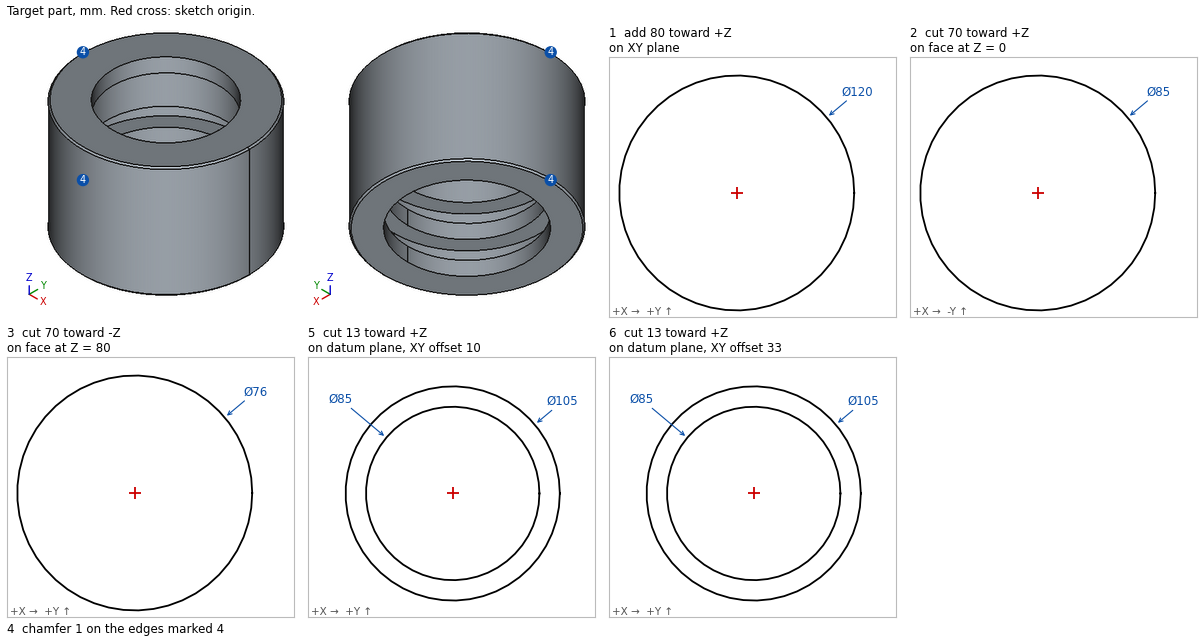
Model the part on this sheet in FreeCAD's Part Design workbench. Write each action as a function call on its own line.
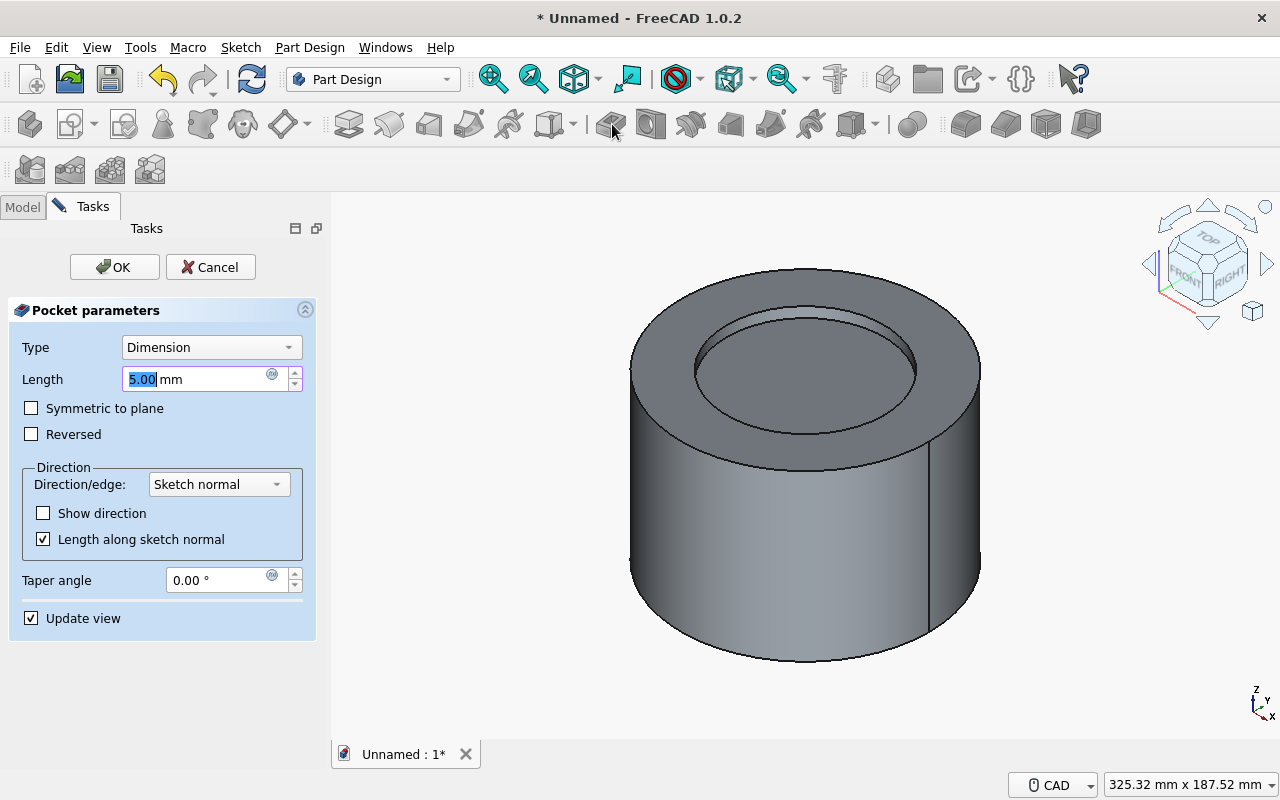
text(70)
key(Tab)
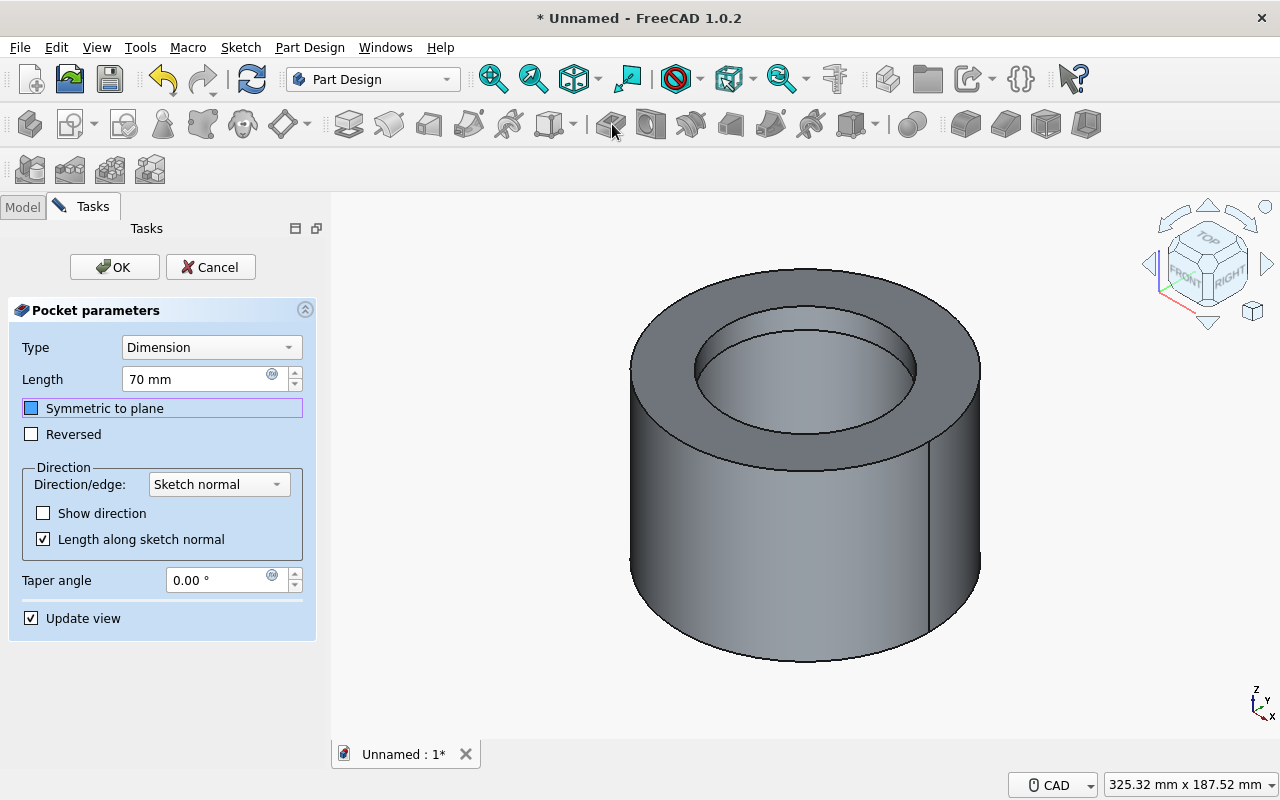
click(115, 267)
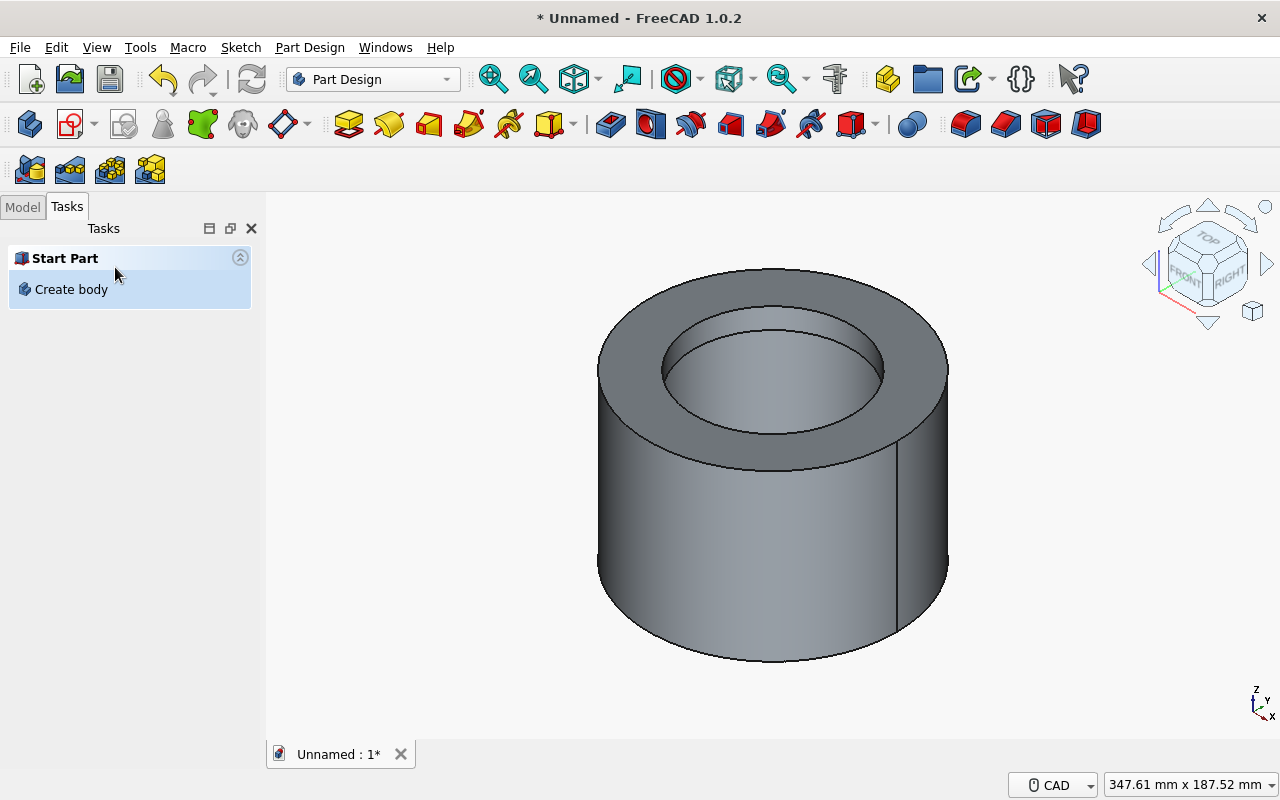
click(617, 415)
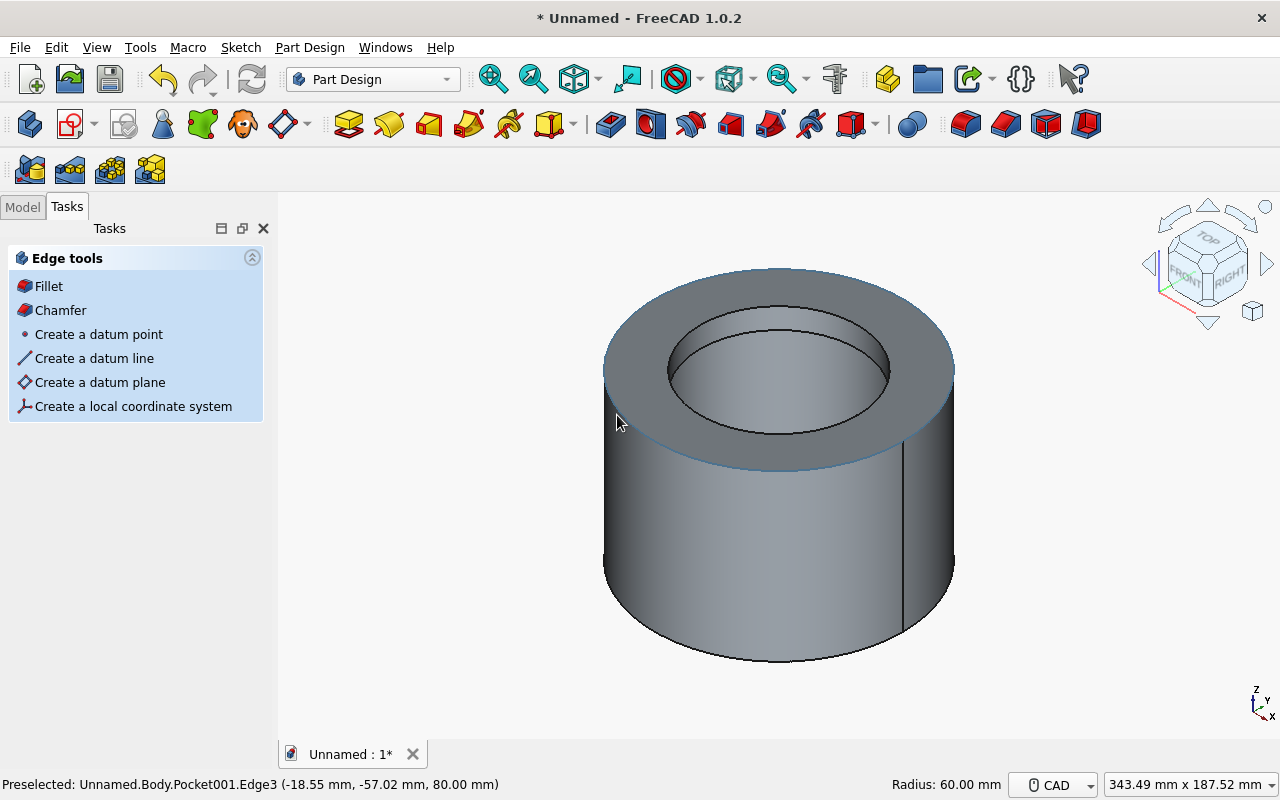
key(2)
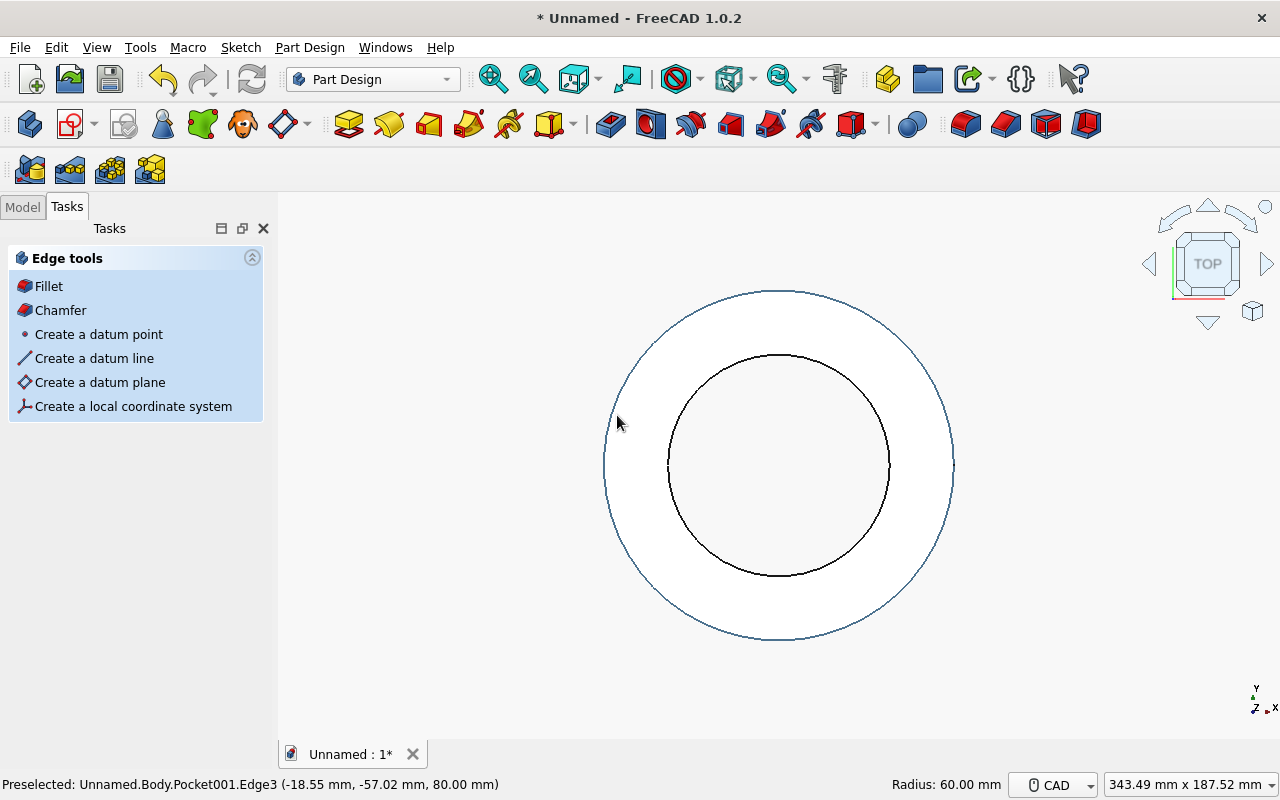
key(0)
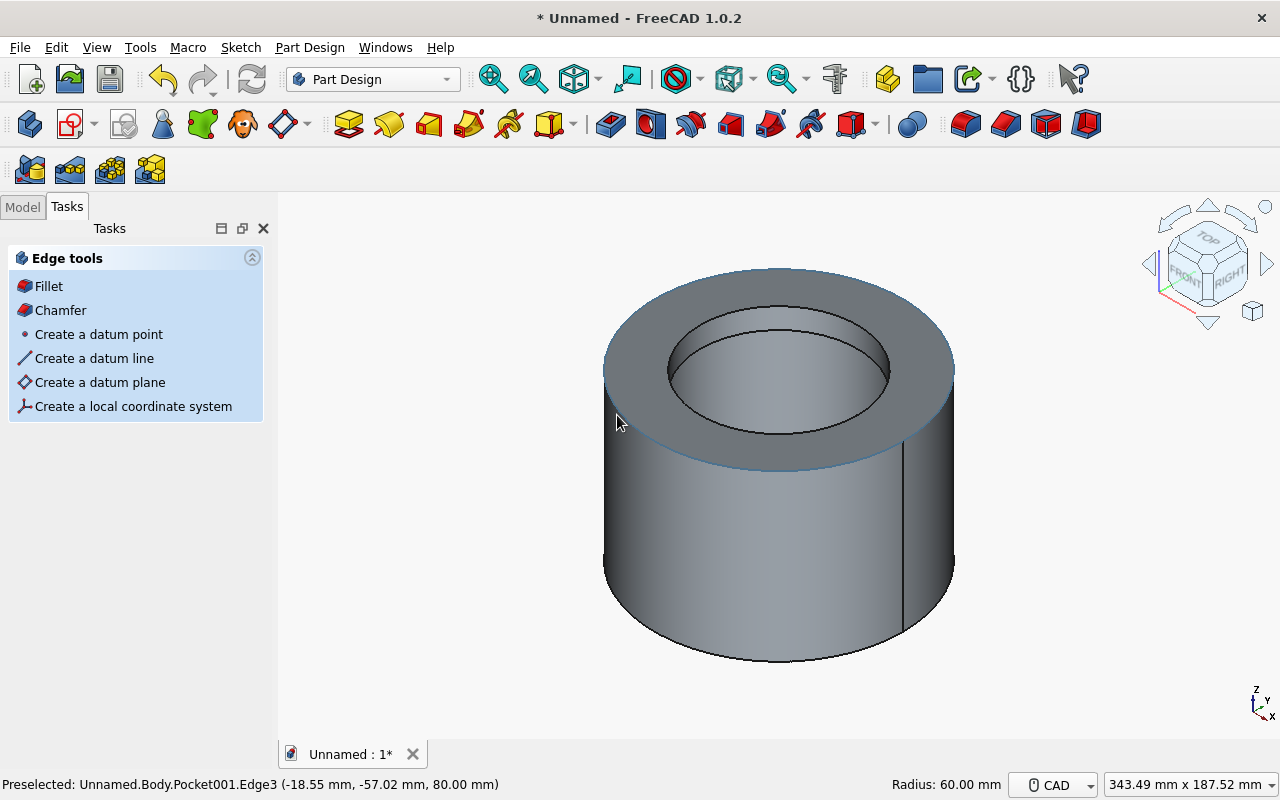
key(1)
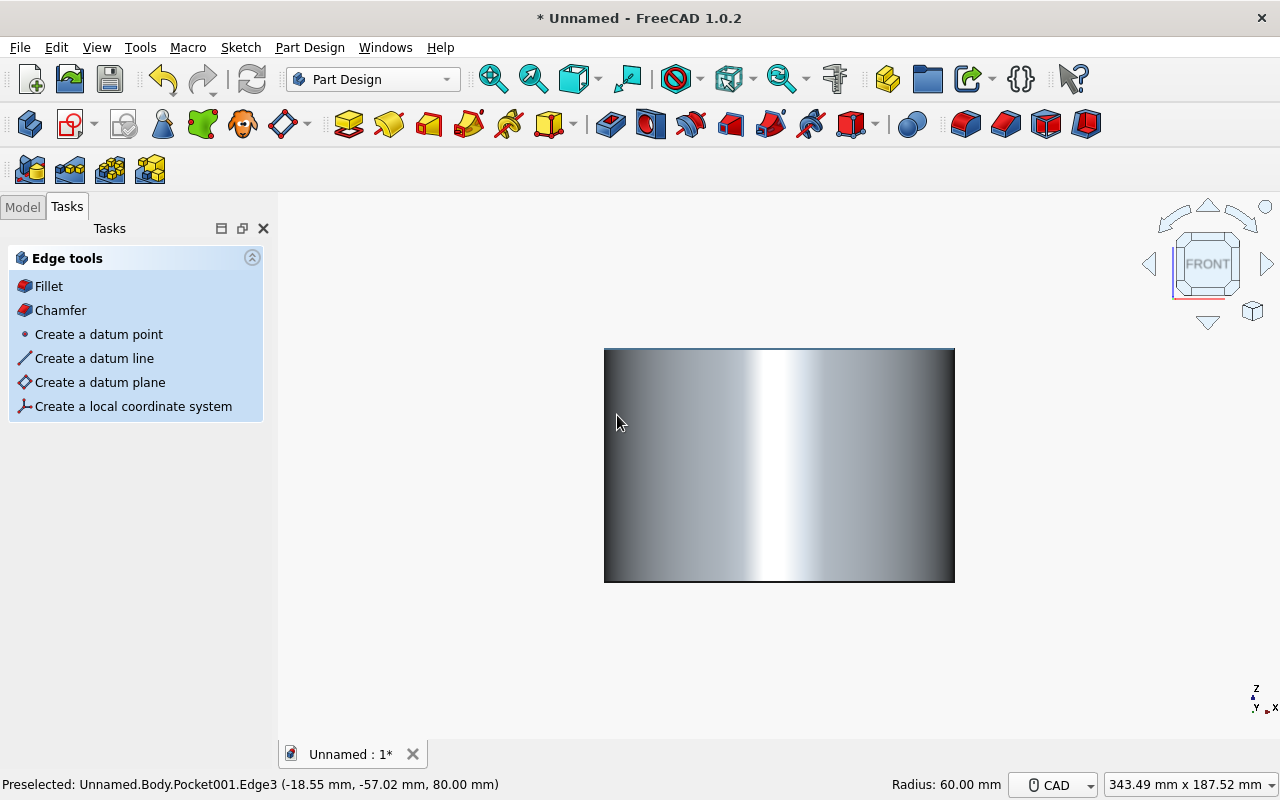
click(494, 80)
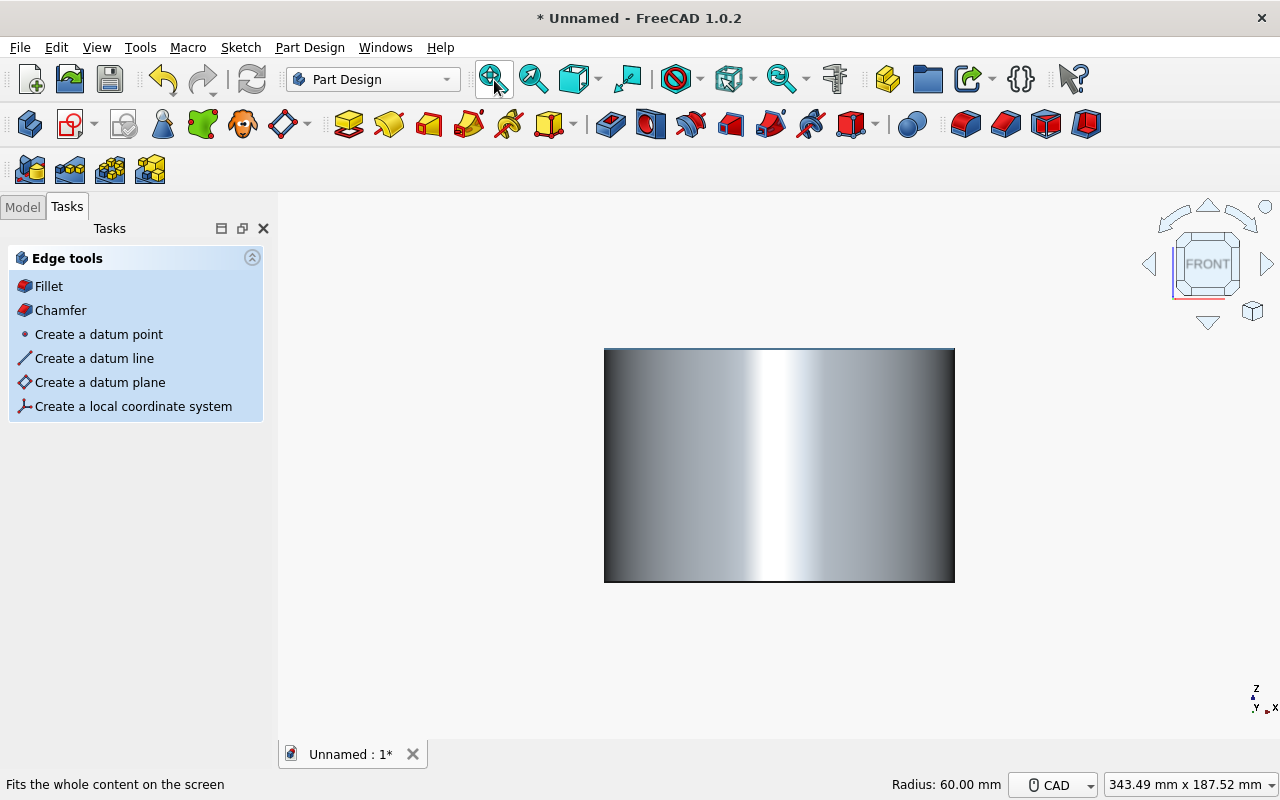
click(637, 581, ctrl)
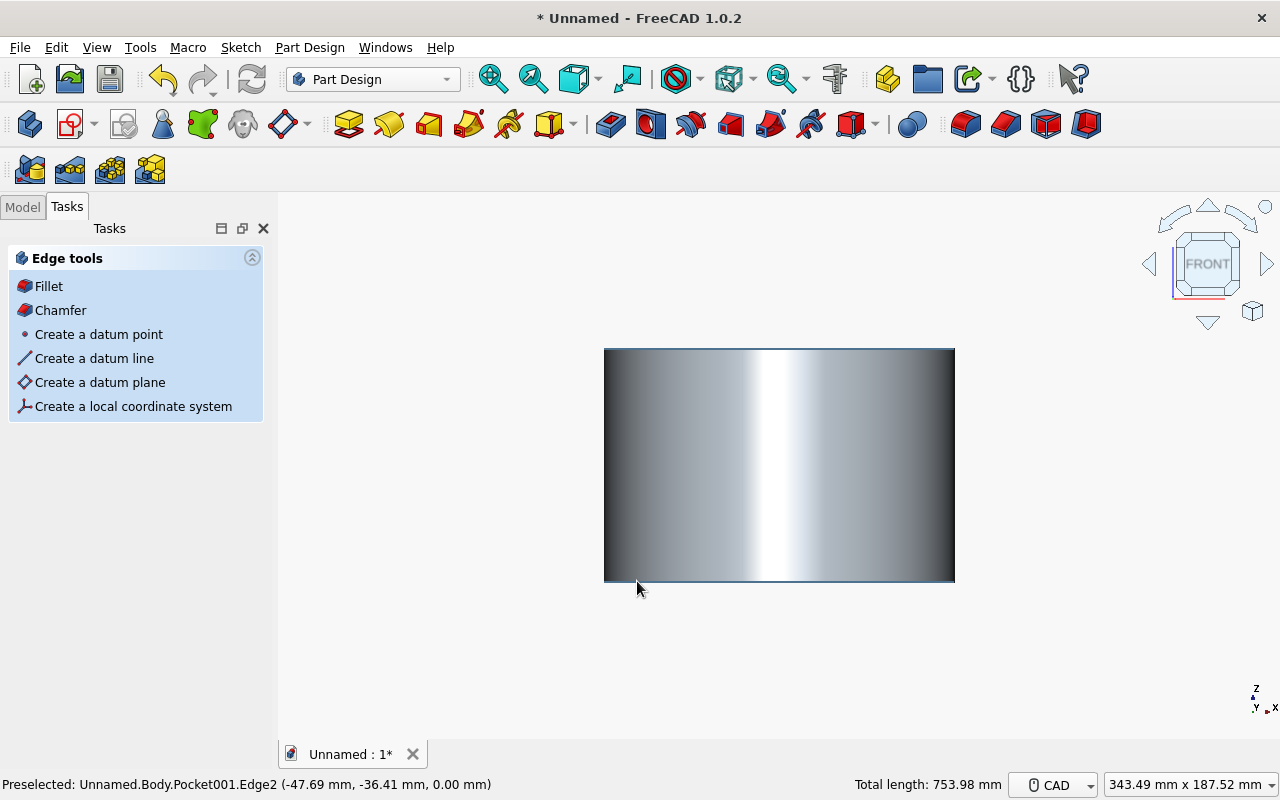
click(1006, 124)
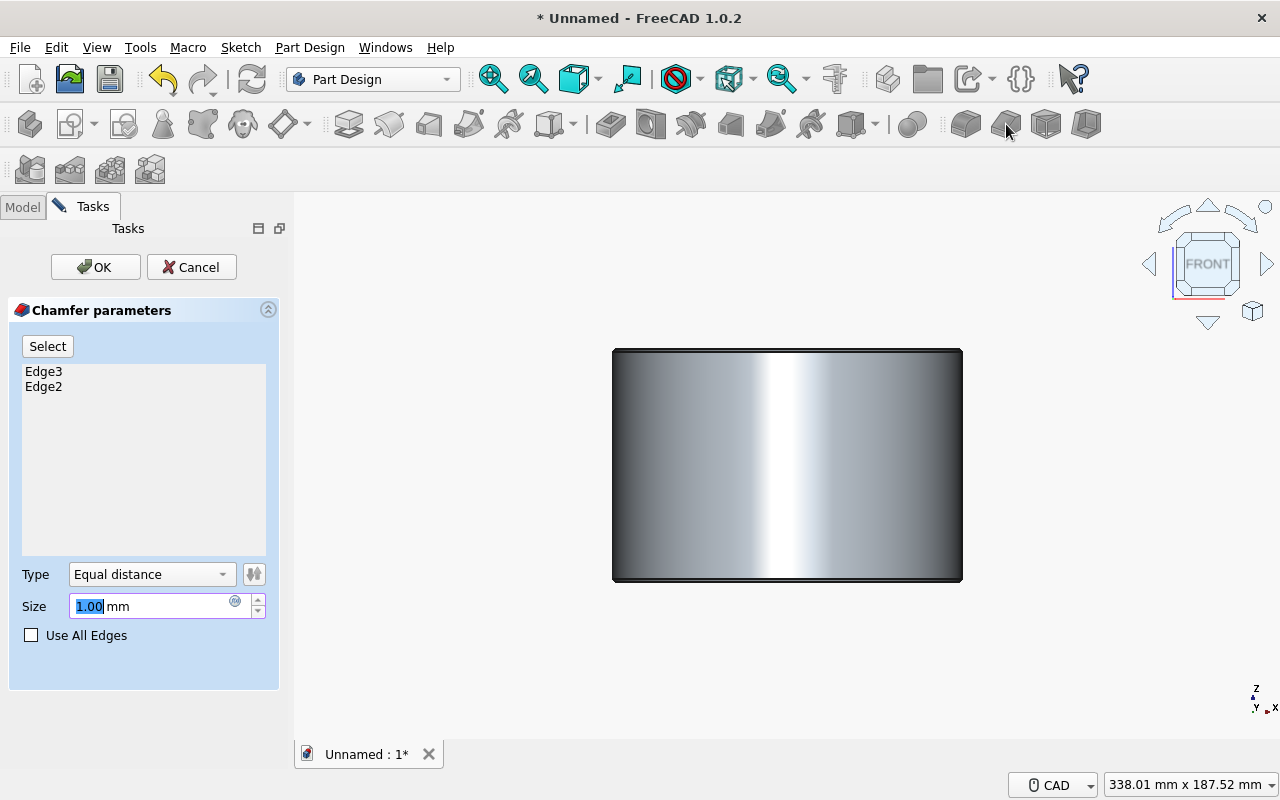
text(1)
key(Tab)